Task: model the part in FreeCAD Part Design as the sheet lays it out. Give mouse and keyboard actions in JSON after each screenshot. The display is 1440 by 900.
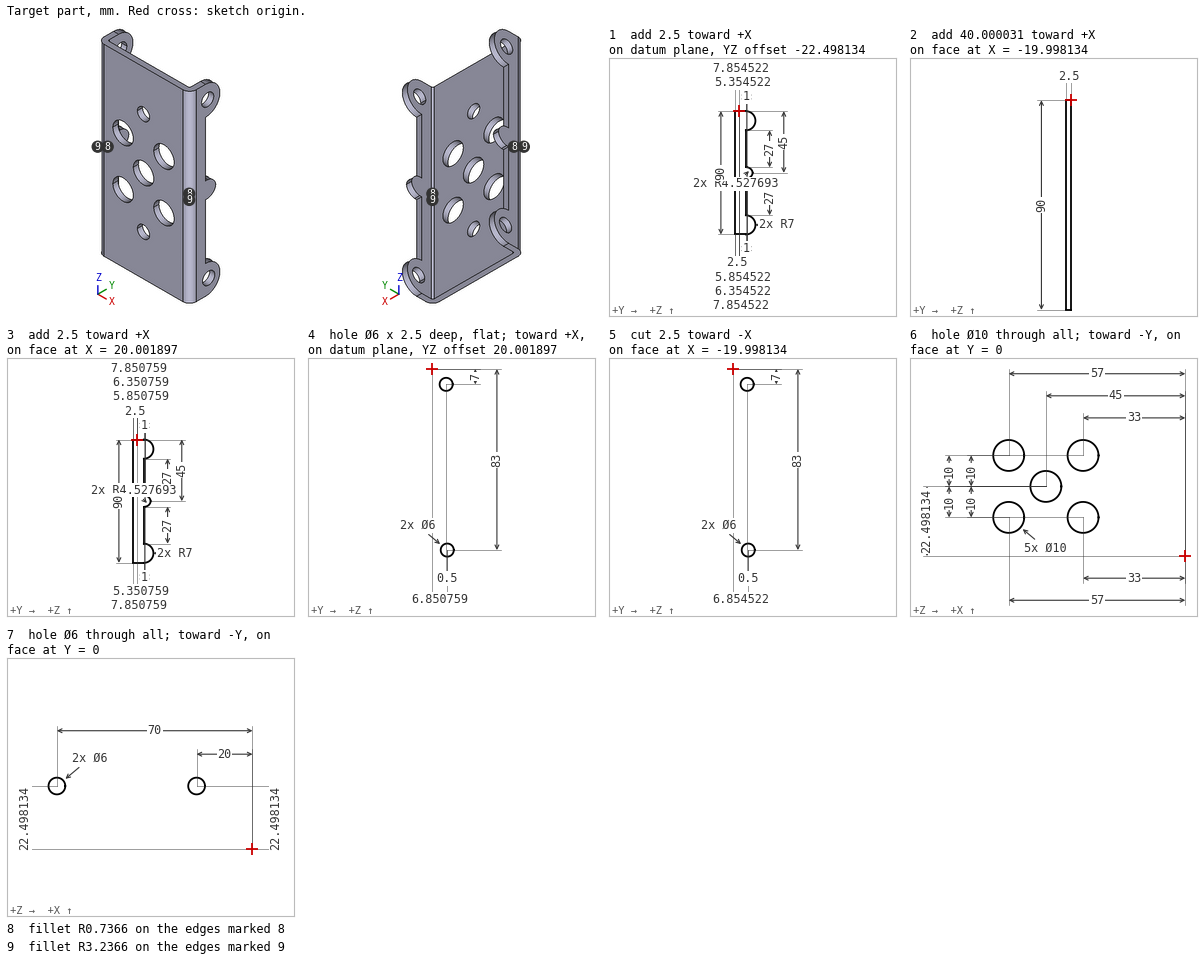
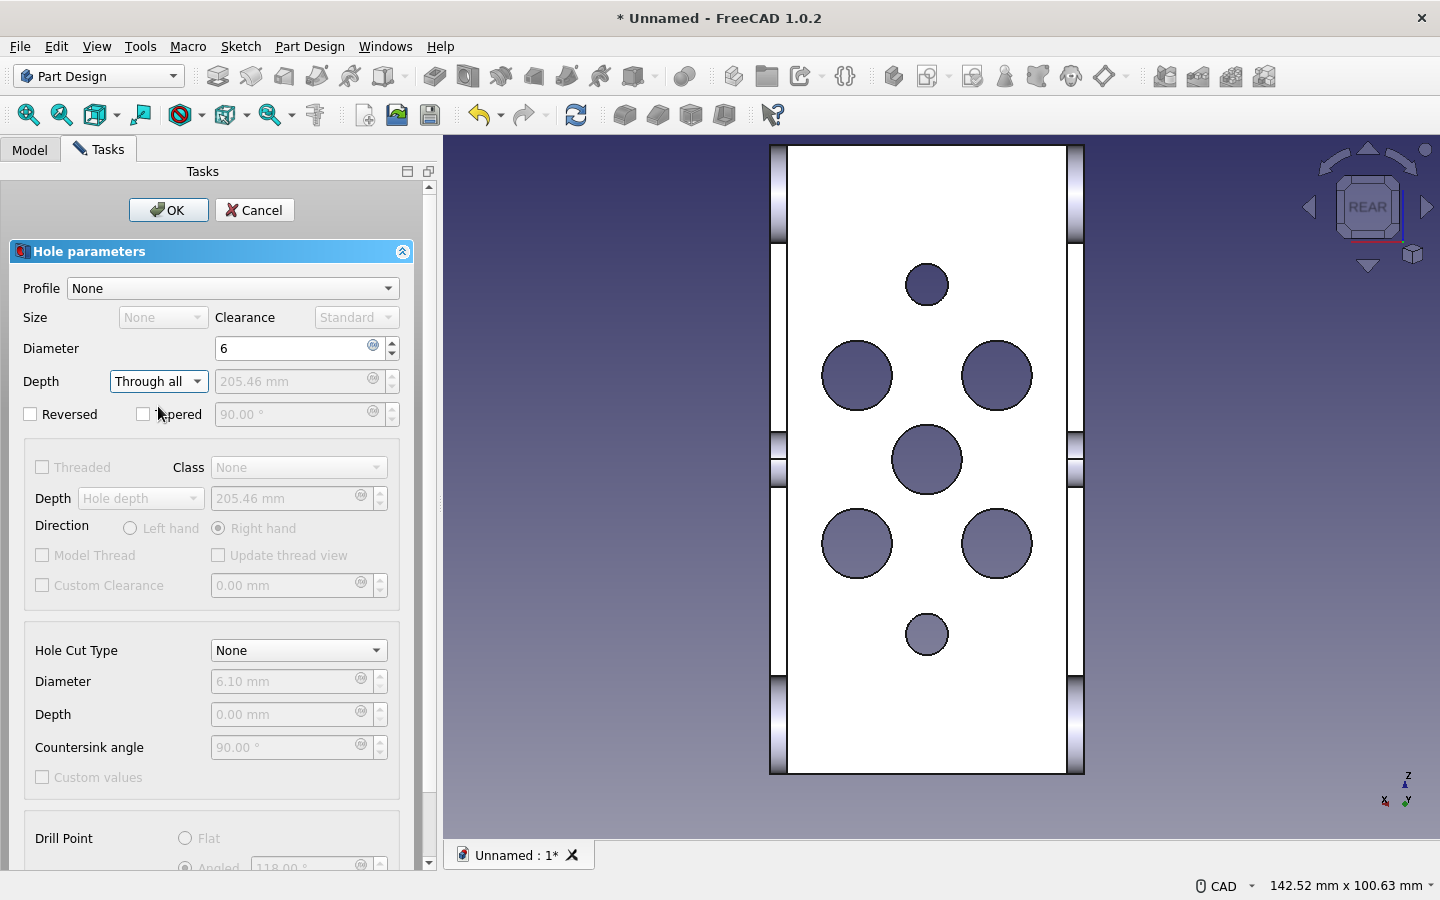
{"action": "left_click", "coordinate": [169, 210]}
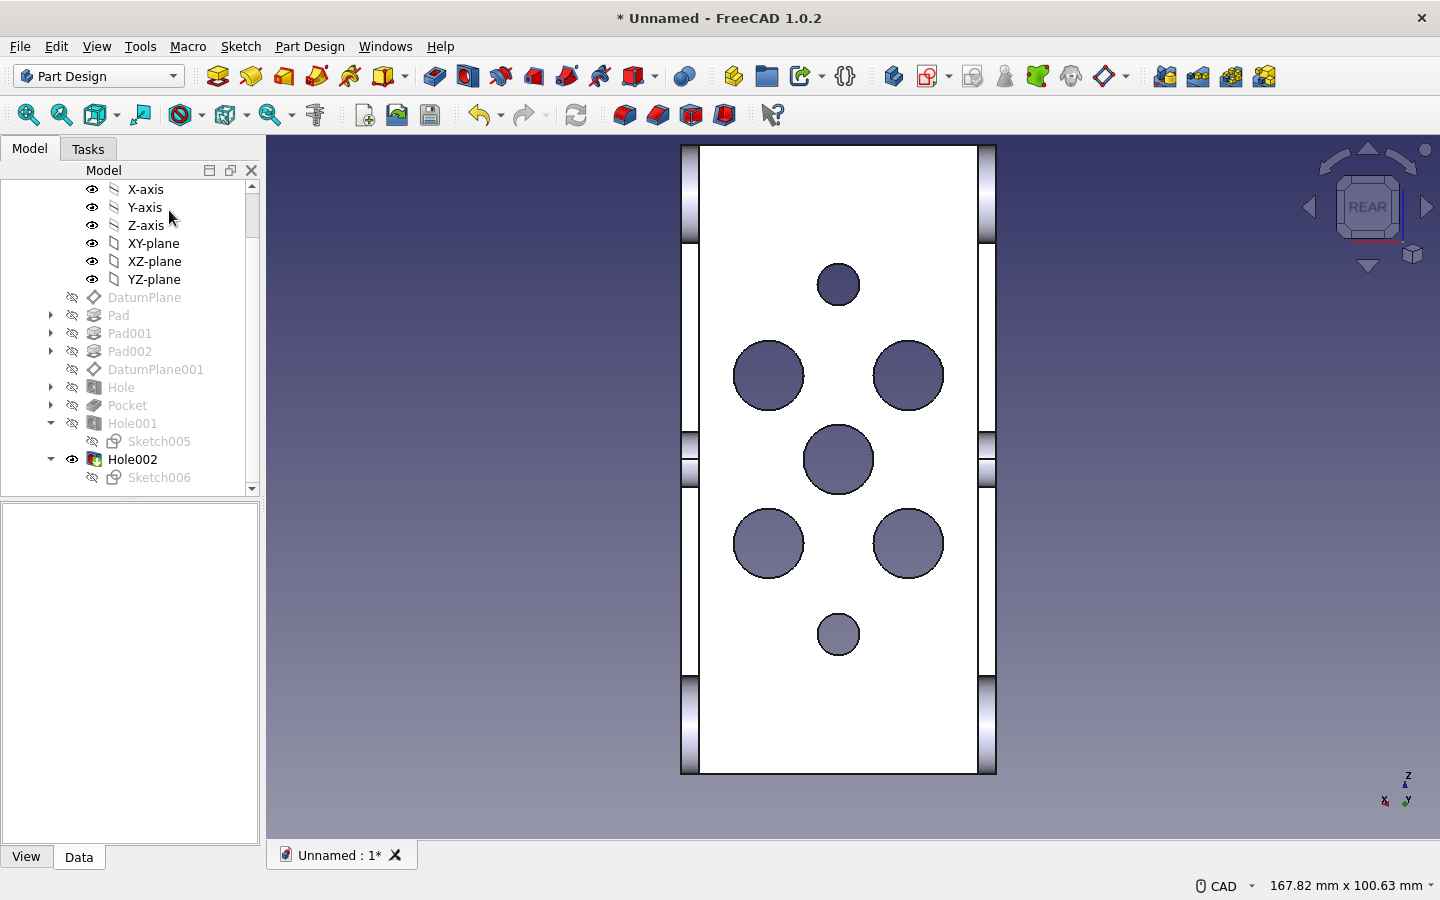
{"action": "key", "text": "0"}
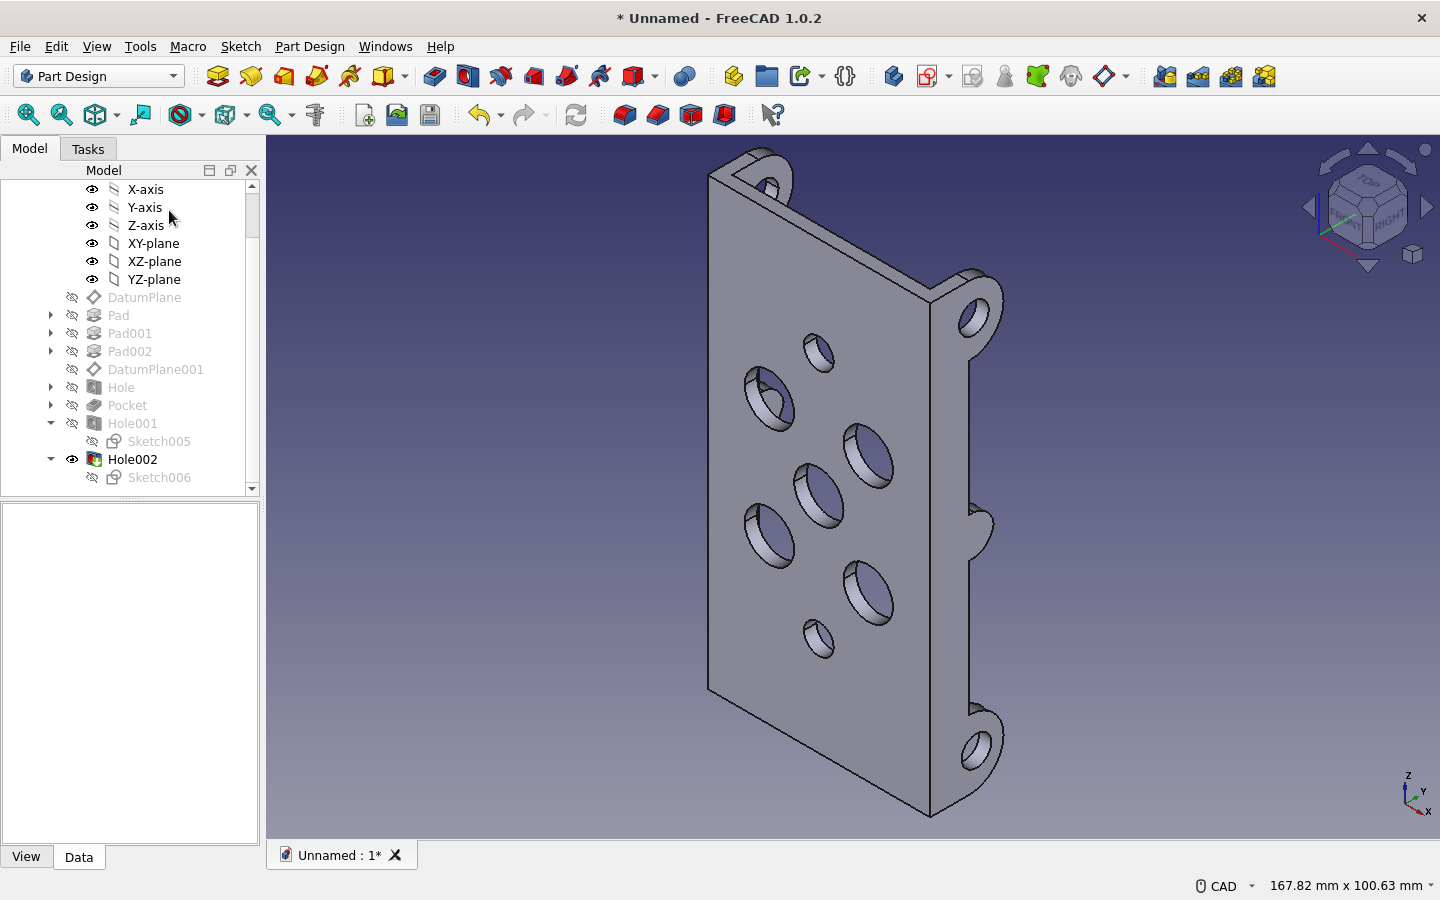
{"action": "key", "text": "v f"}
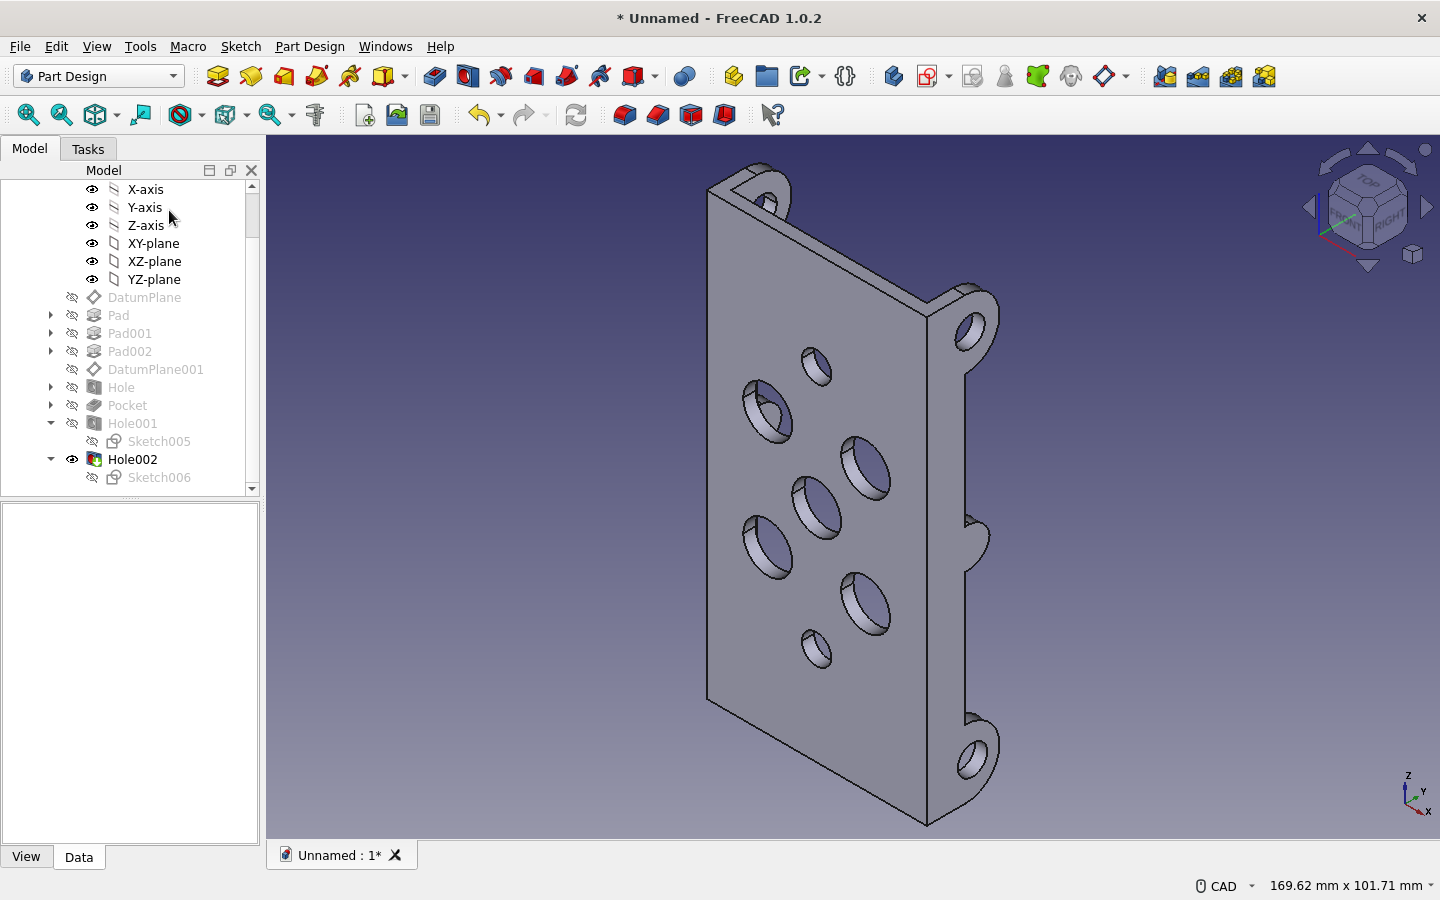
{"action": "key", "text": "2"}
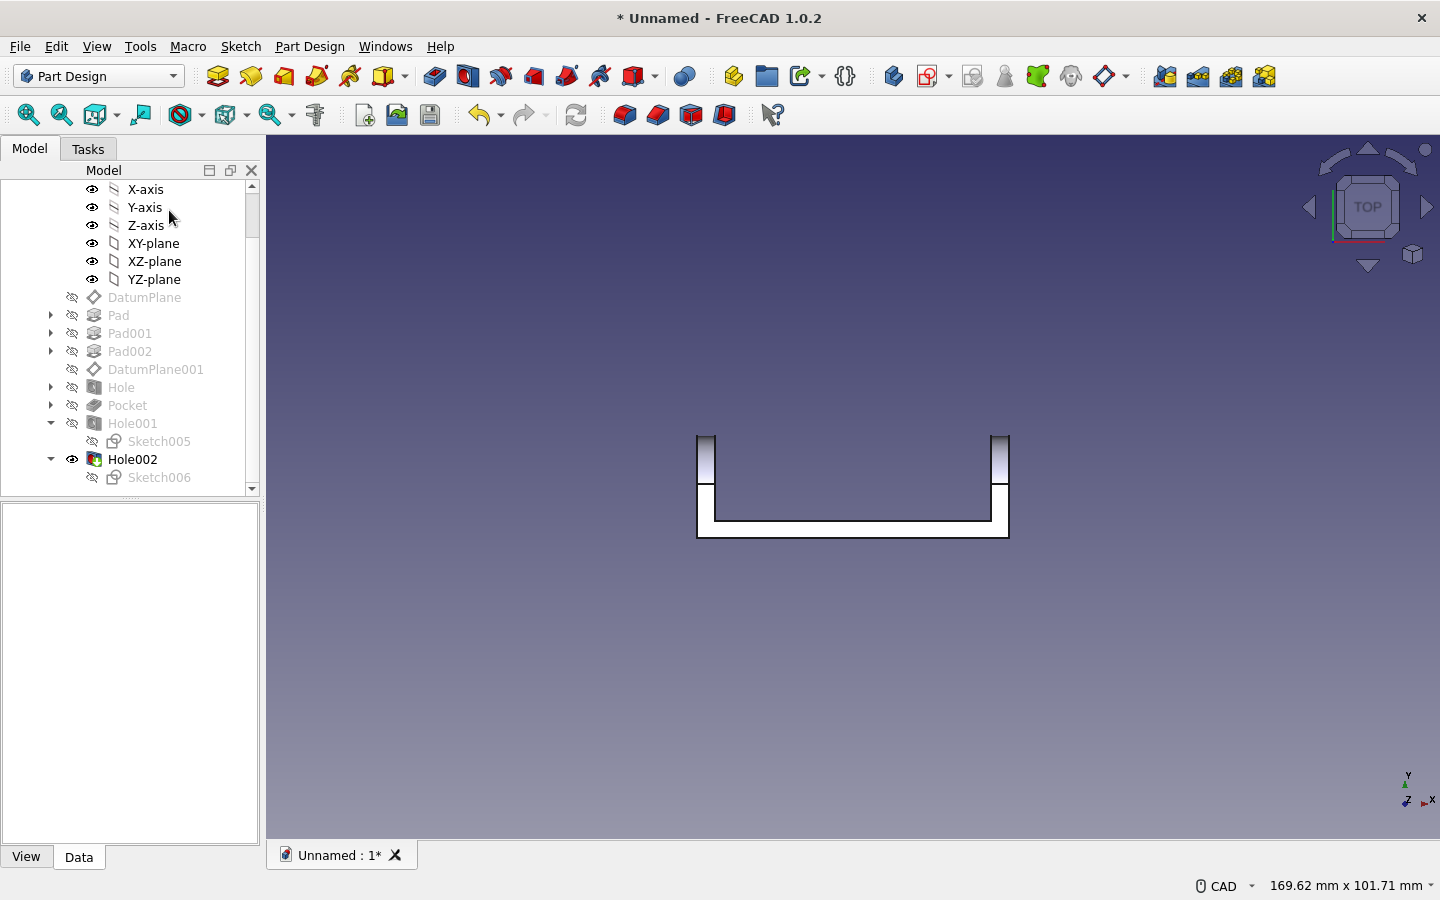
{"action": "left_click", "coordinate": [29, 116]}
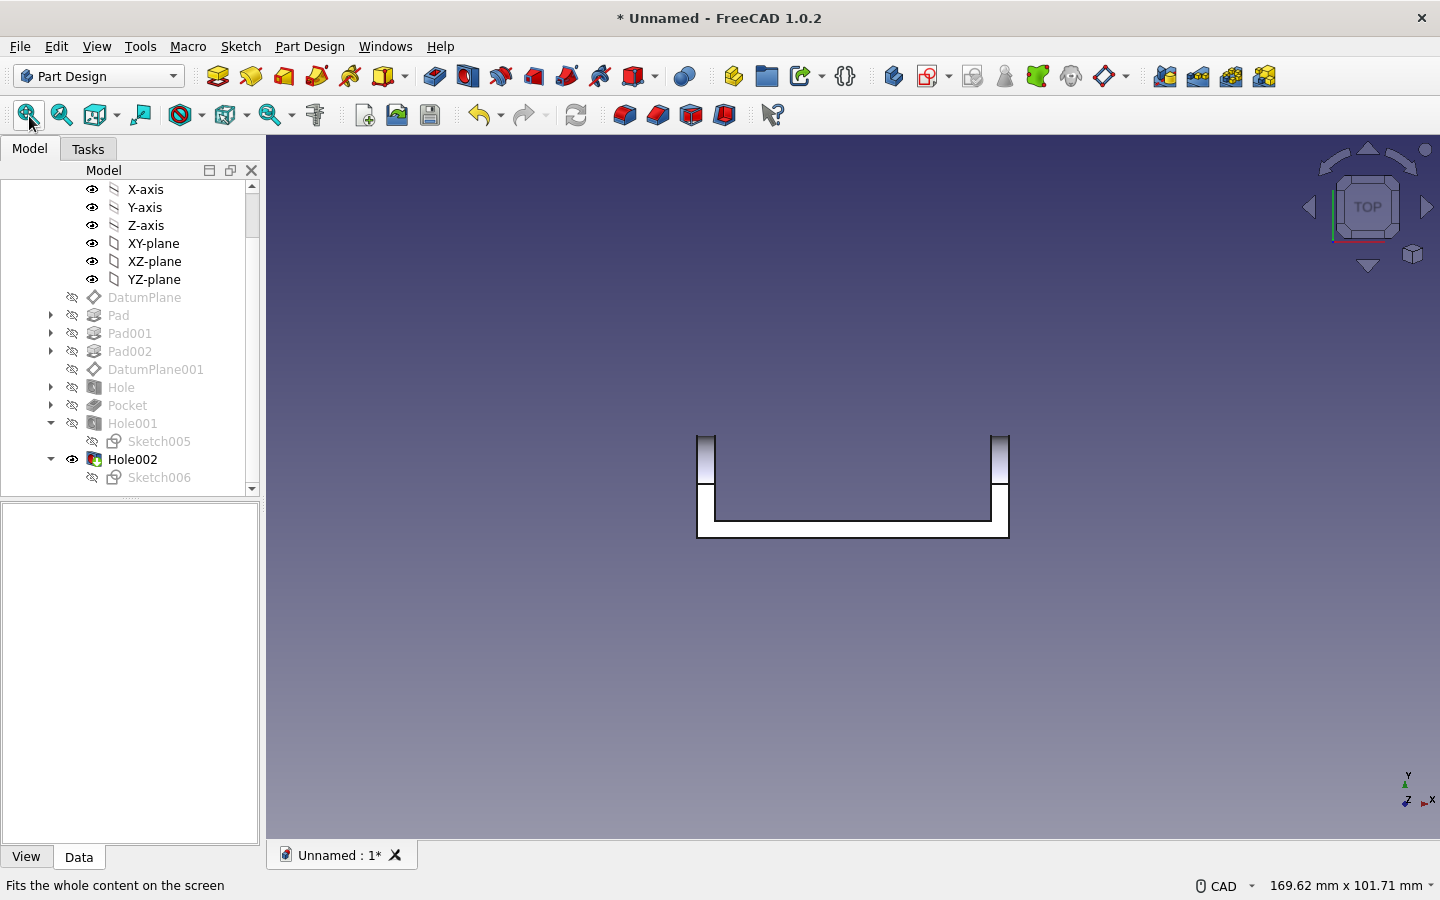
{"action": "key", "text": "1"}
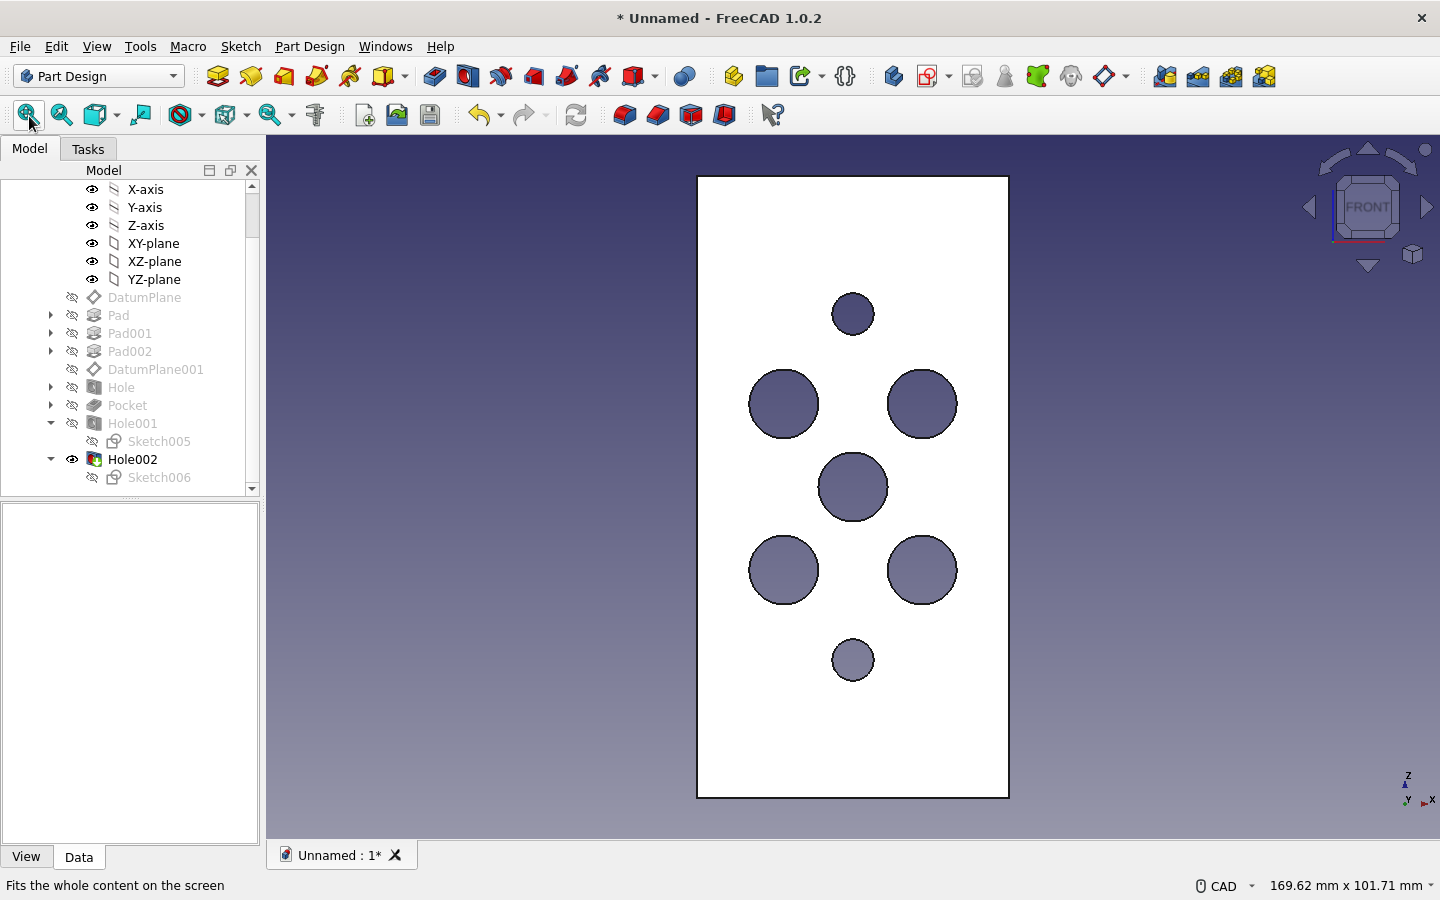
{"action": "key", "text": "3"}